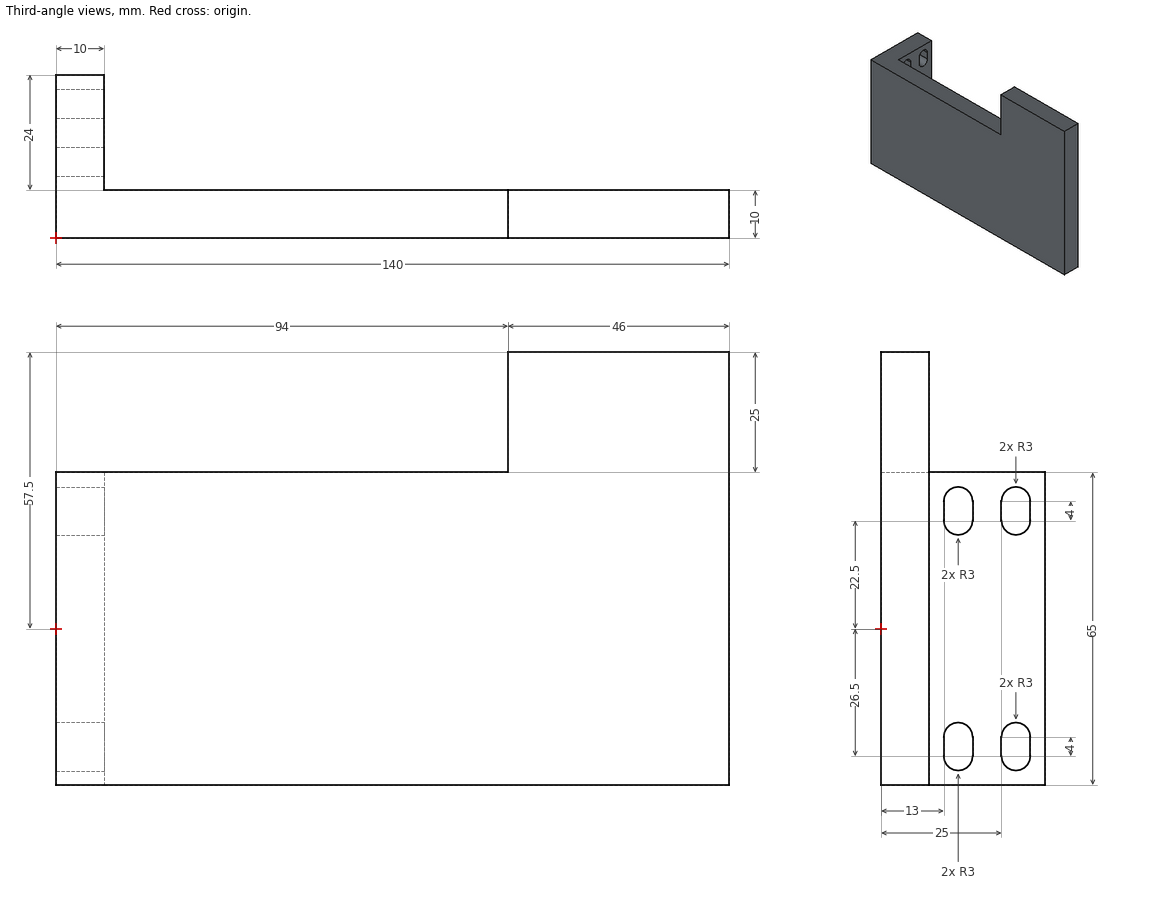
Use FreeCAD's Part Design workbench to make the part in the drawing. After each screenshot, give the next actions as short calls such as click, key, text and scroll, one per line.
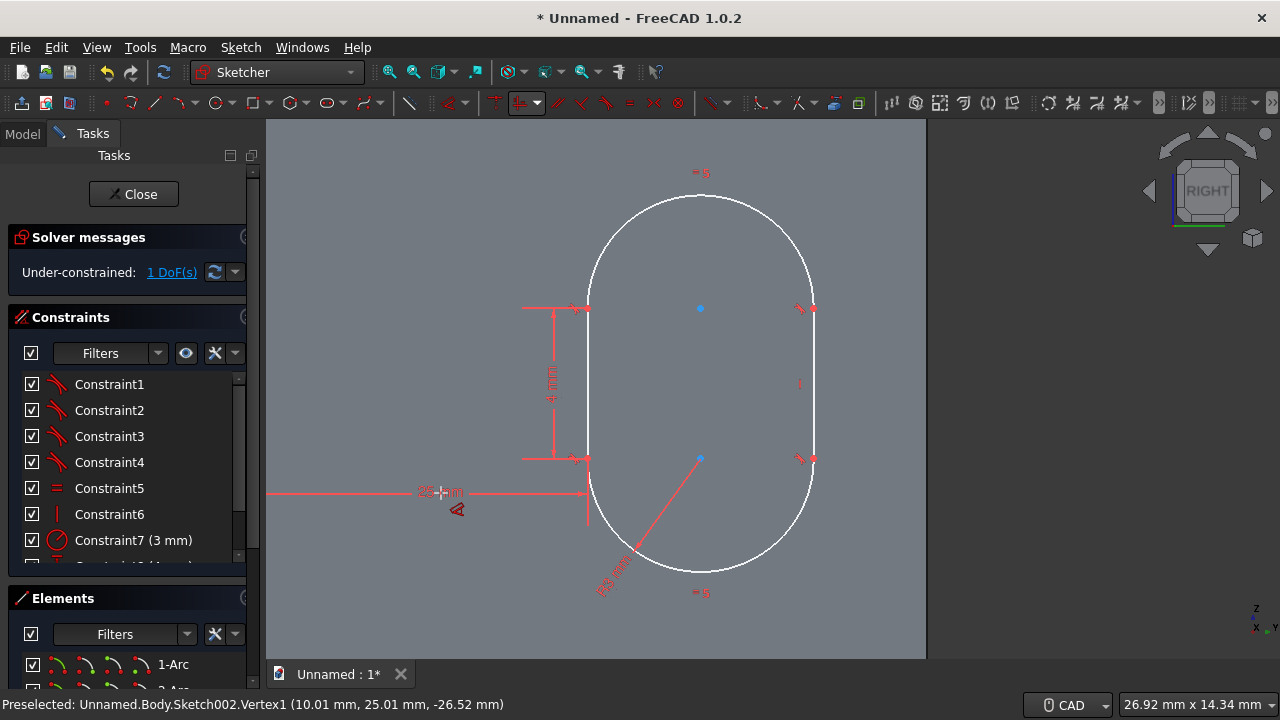
click(588, 459)
click(622, 303)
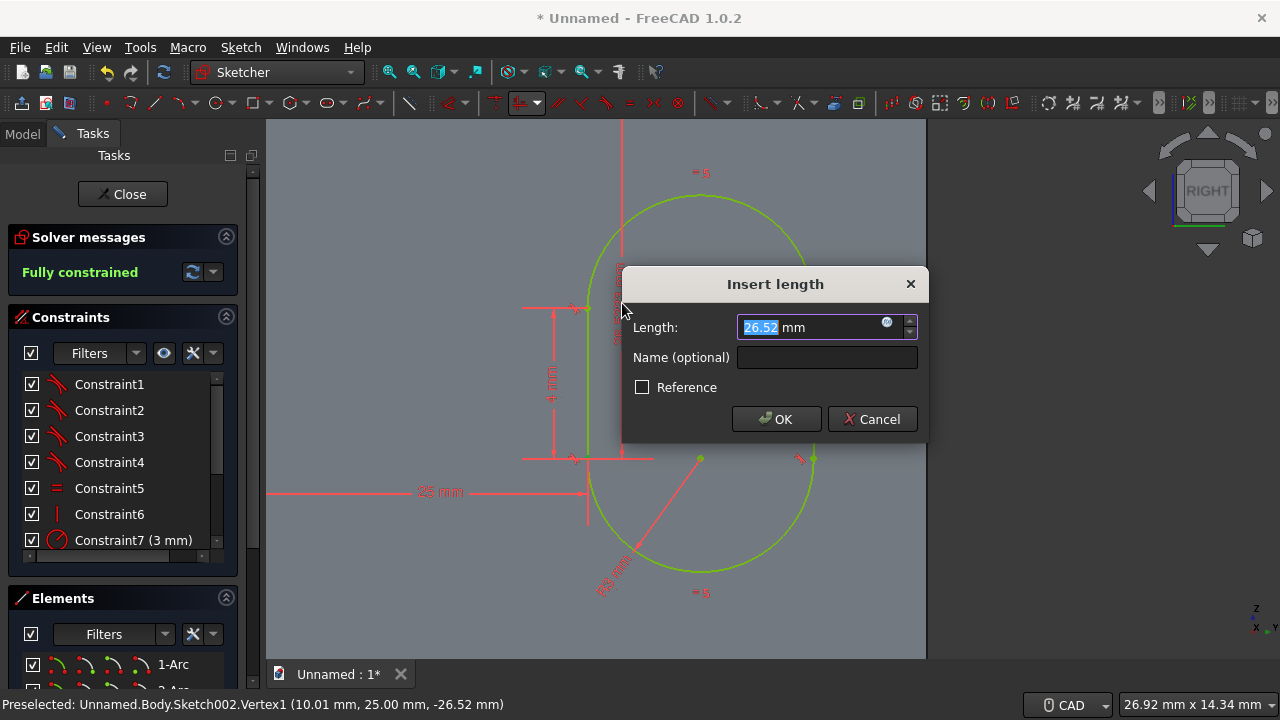
text(26.5)
key(Return)
key(Escape)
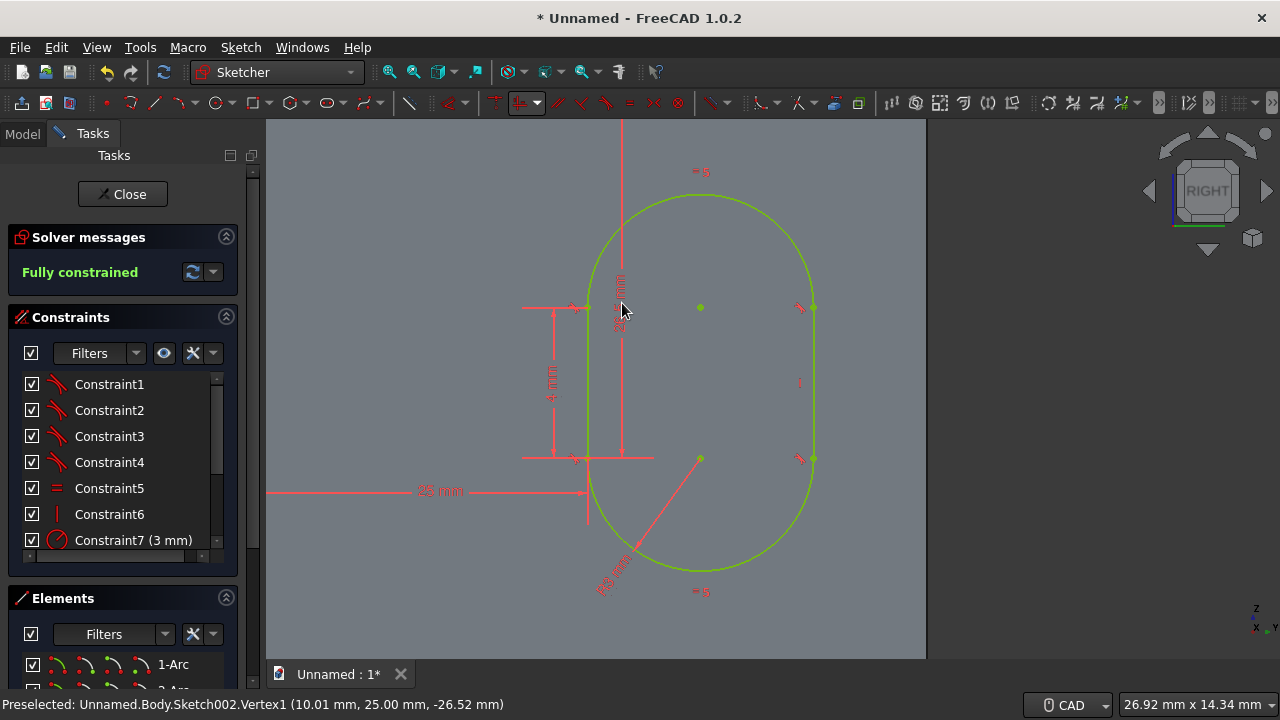
click(123, 194)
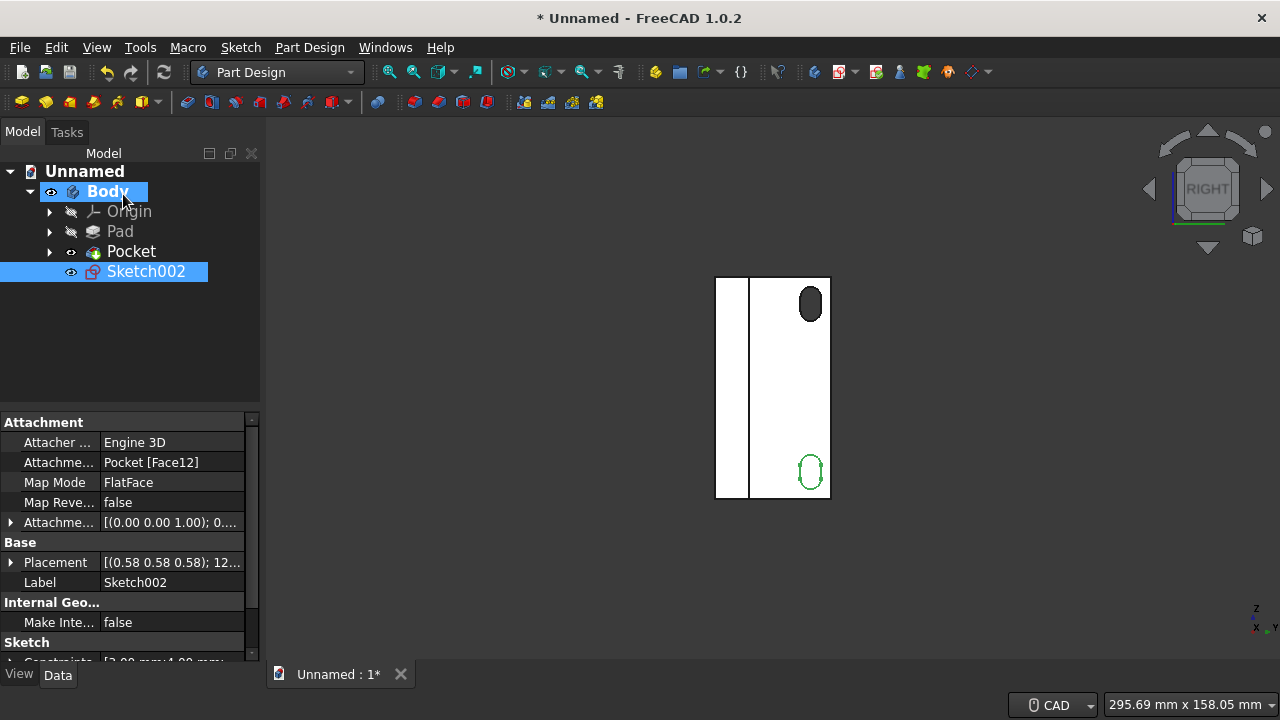
click(188, 102)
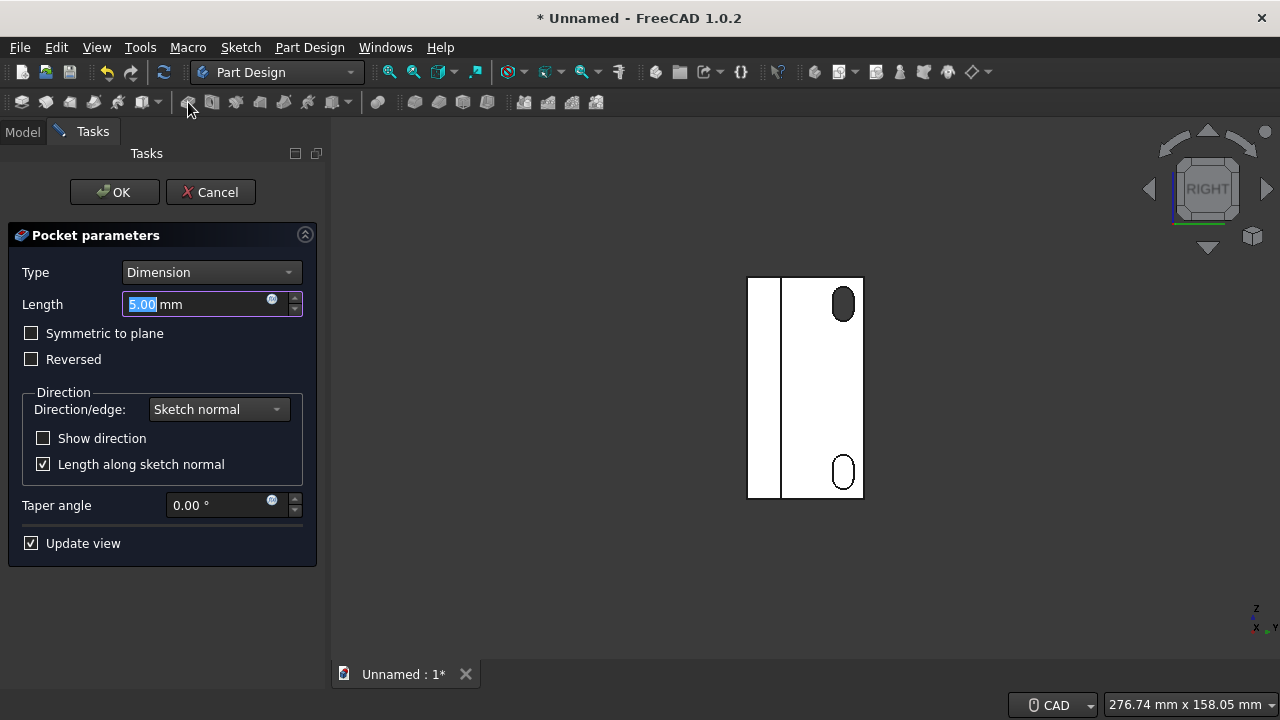
click(212, 272)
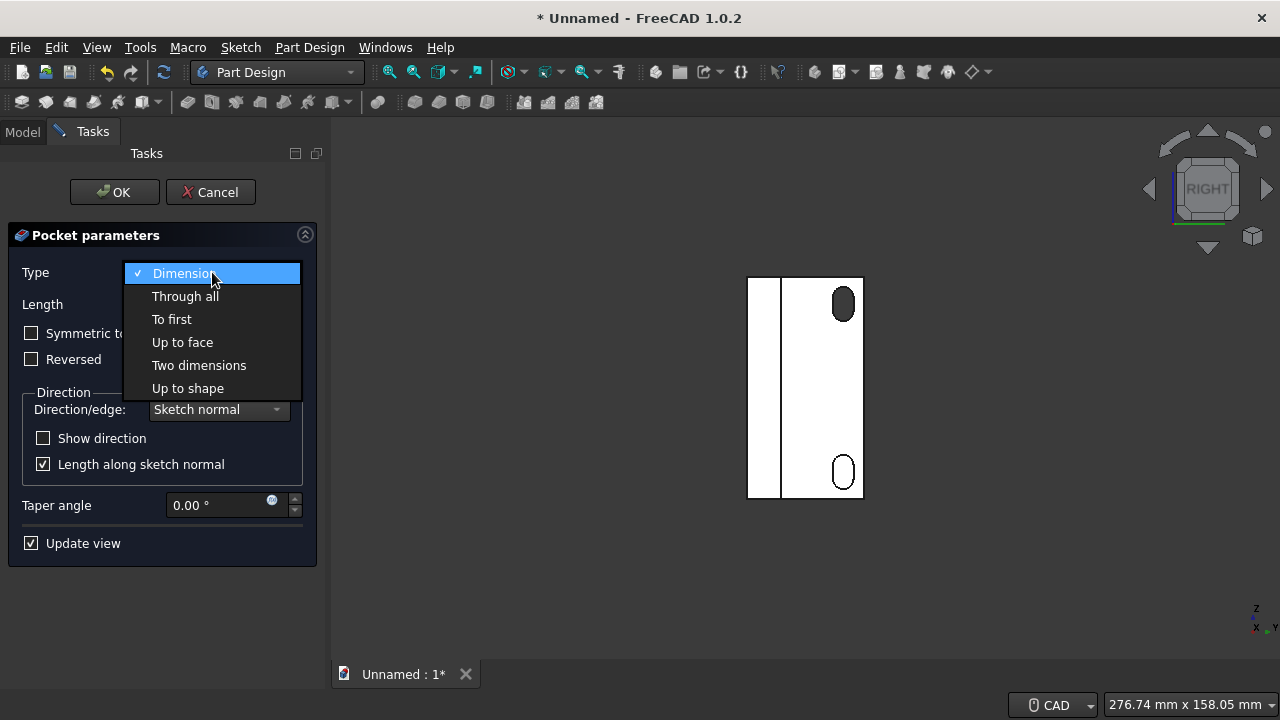
click(212, 320)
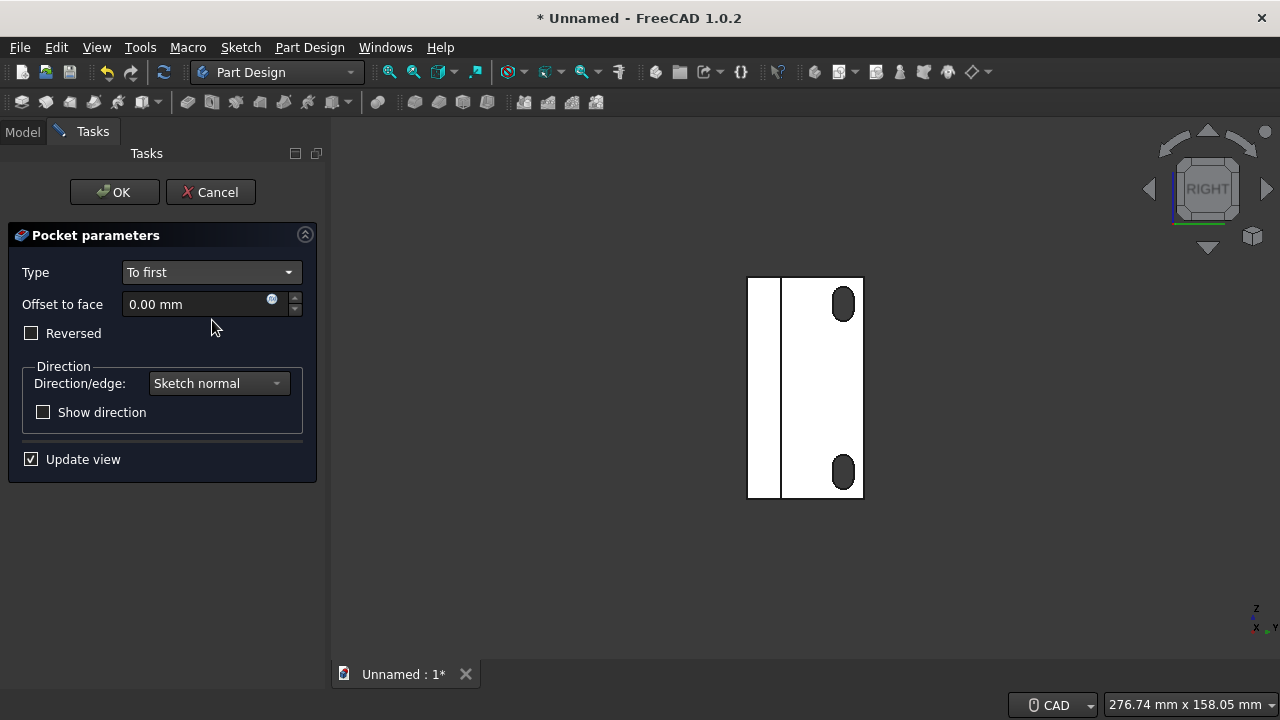
click(115, 192)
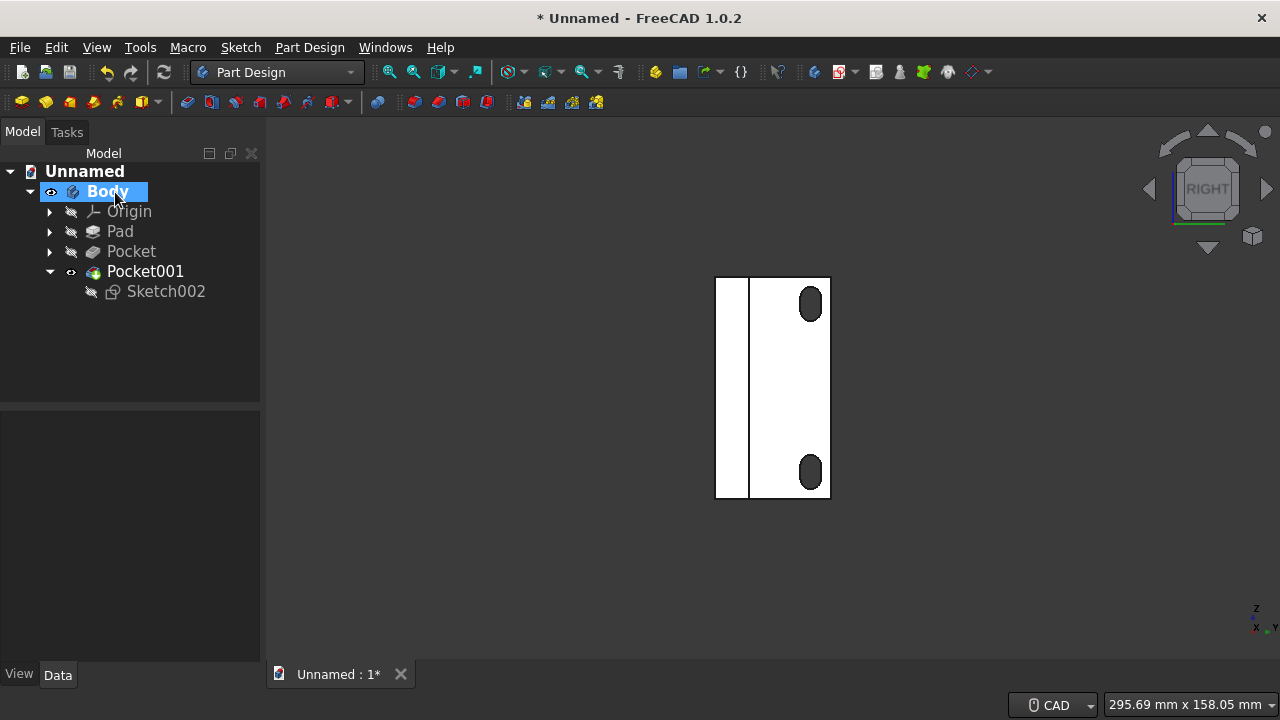
key(v)
key(f)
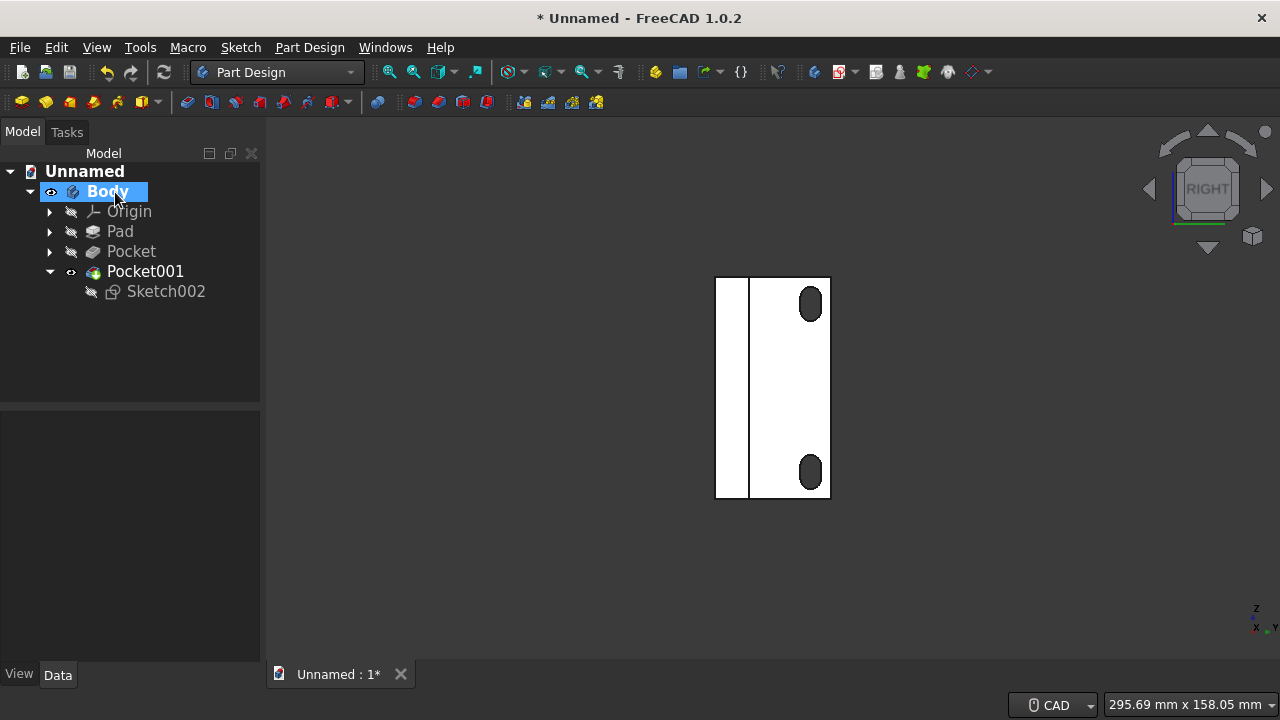
click(790, 387)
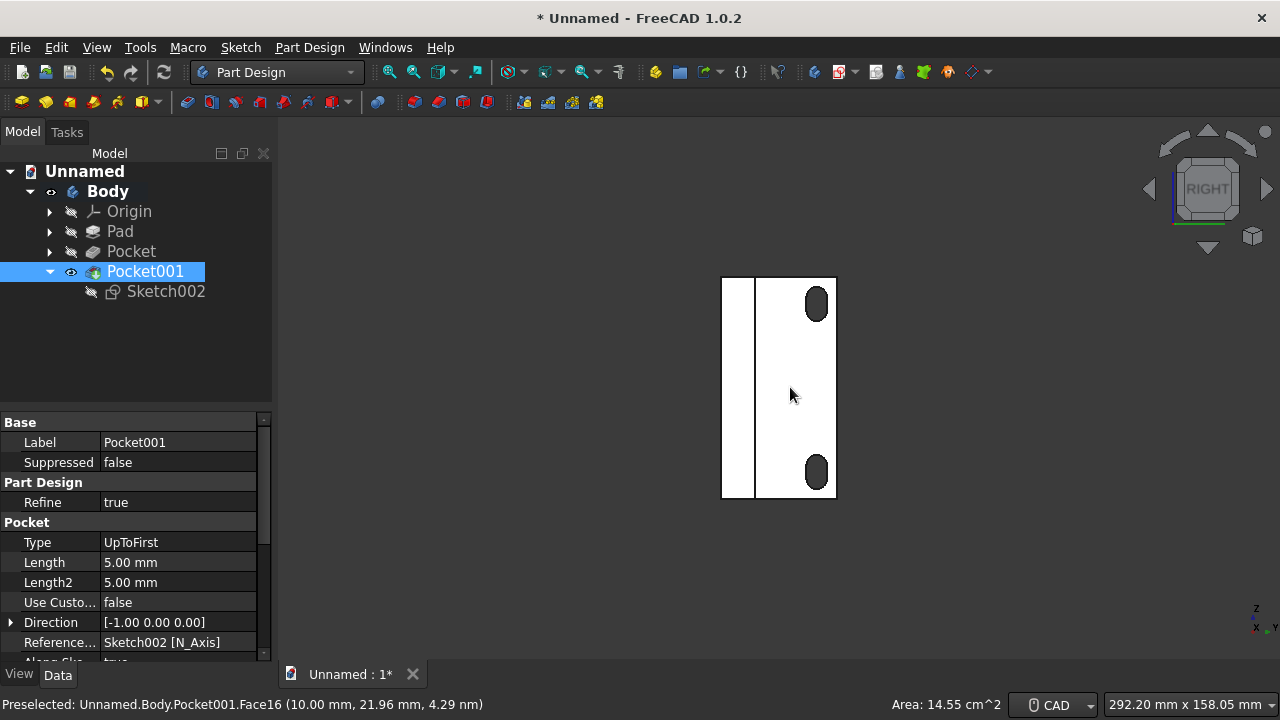
click(840, 72)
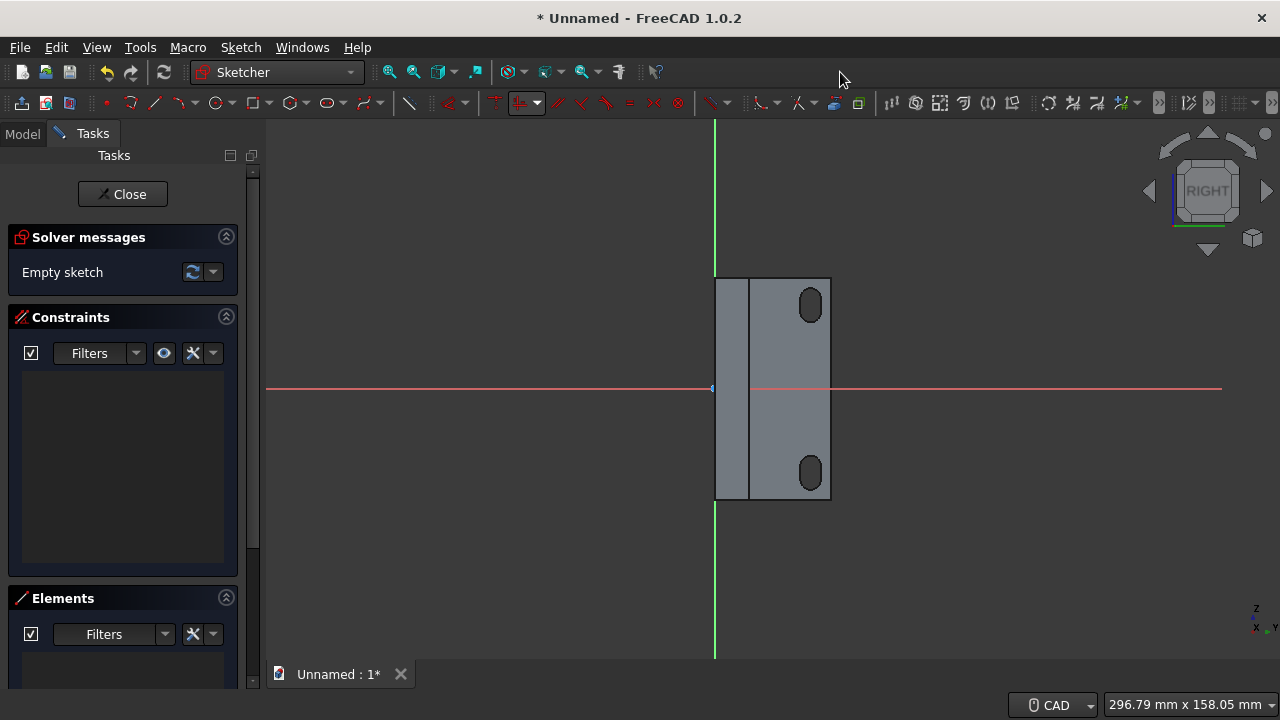
scroll(776, 297, up, 12)